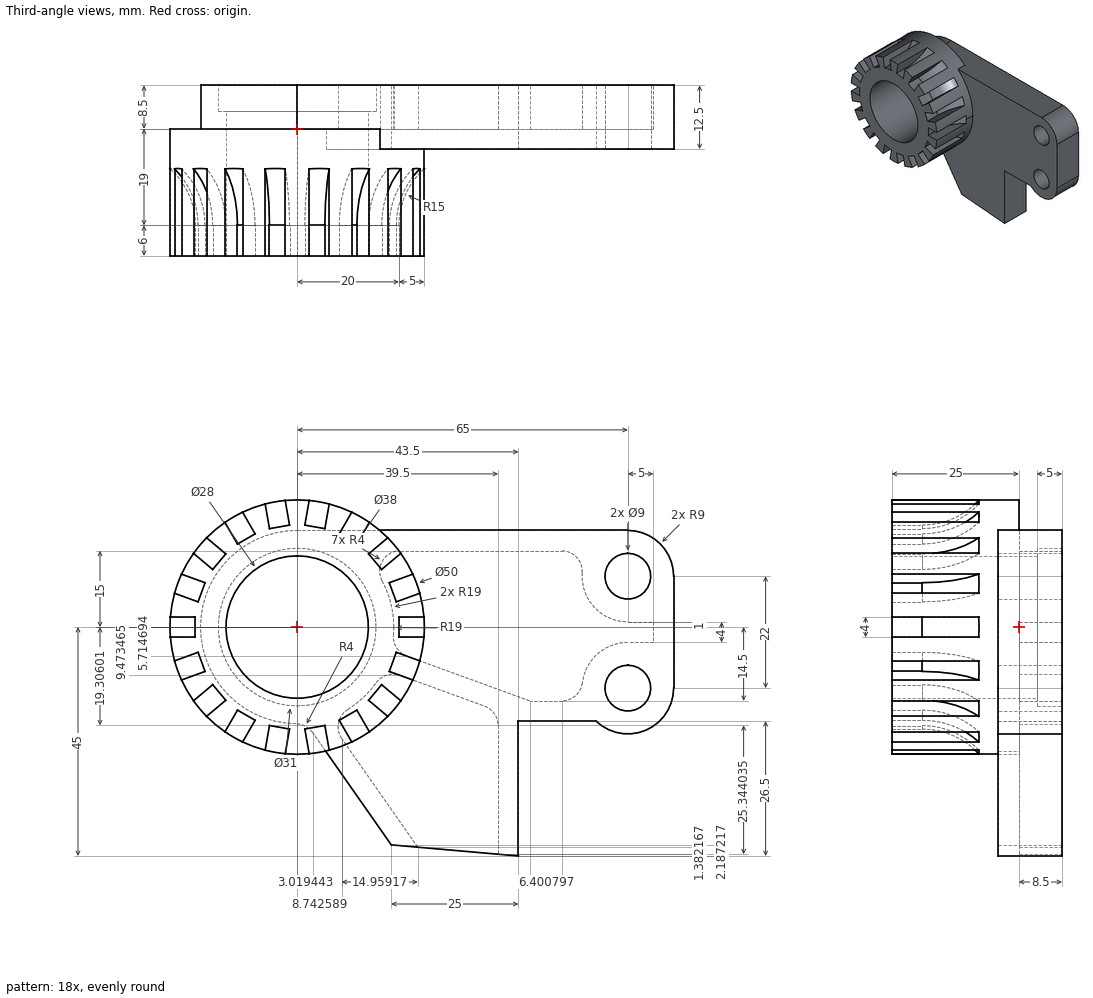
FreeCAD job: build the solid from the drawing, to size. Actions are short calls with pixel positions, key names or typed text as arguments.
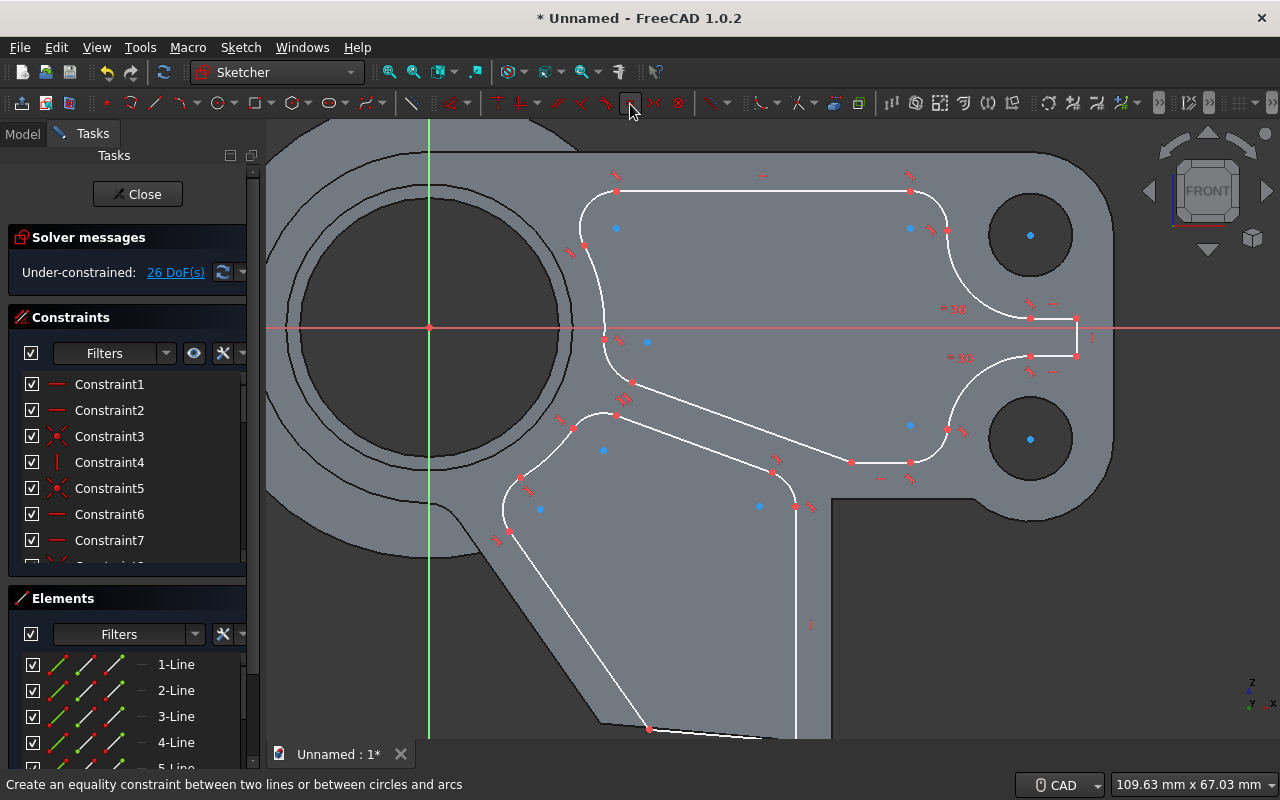
click(944, 213)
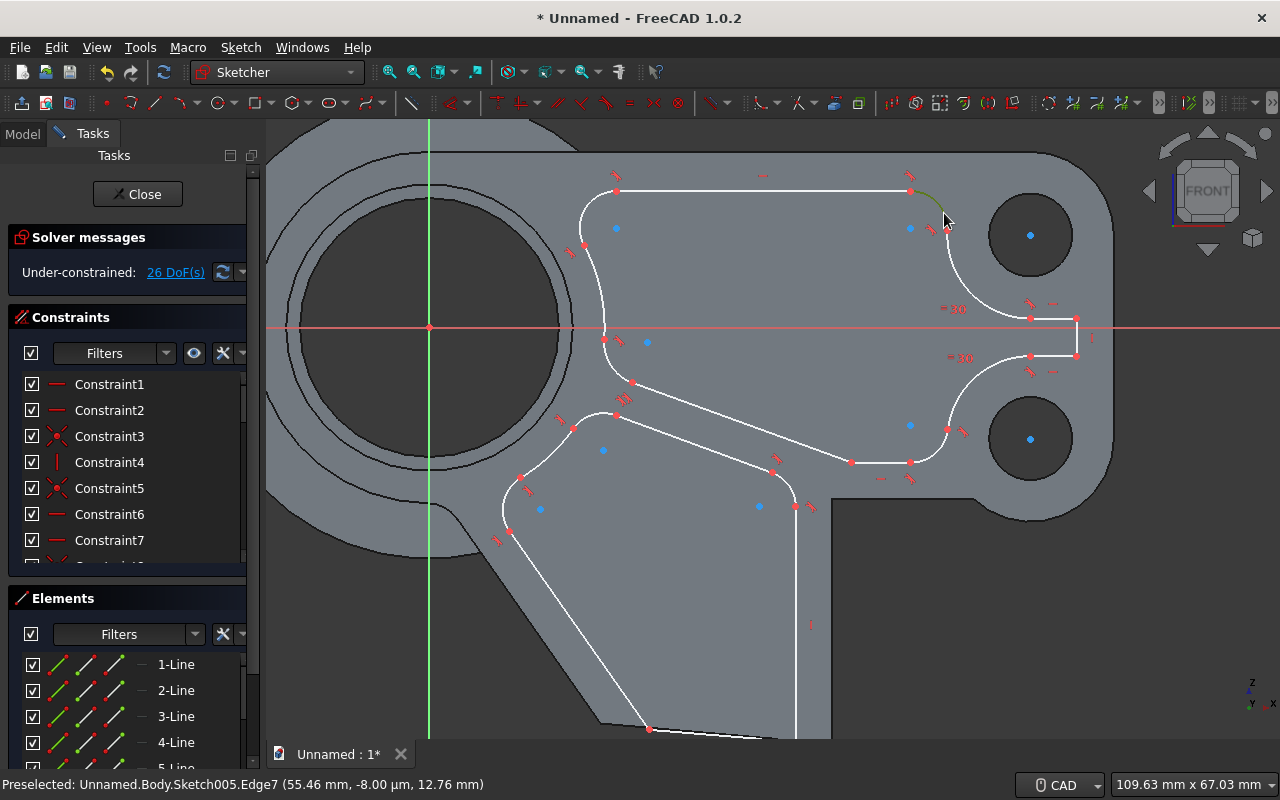
click(927, 459)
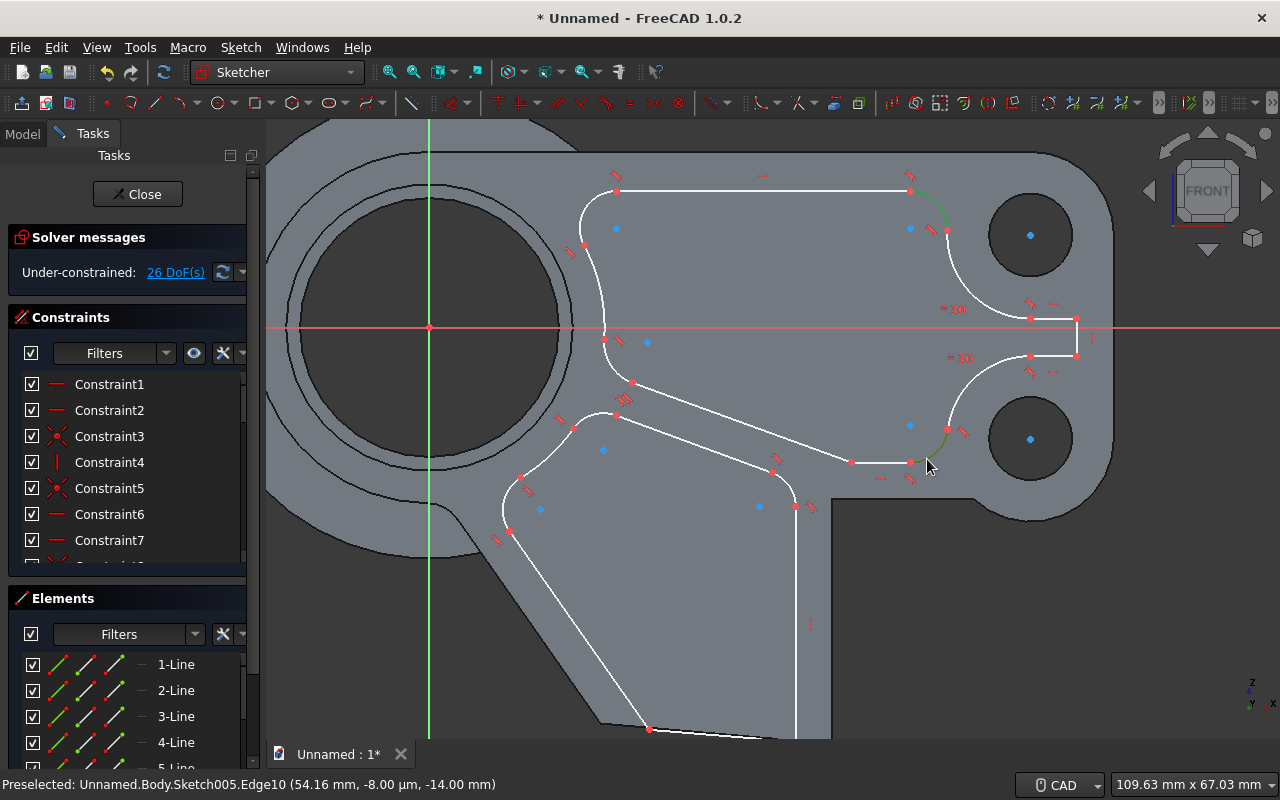
click(606, 356)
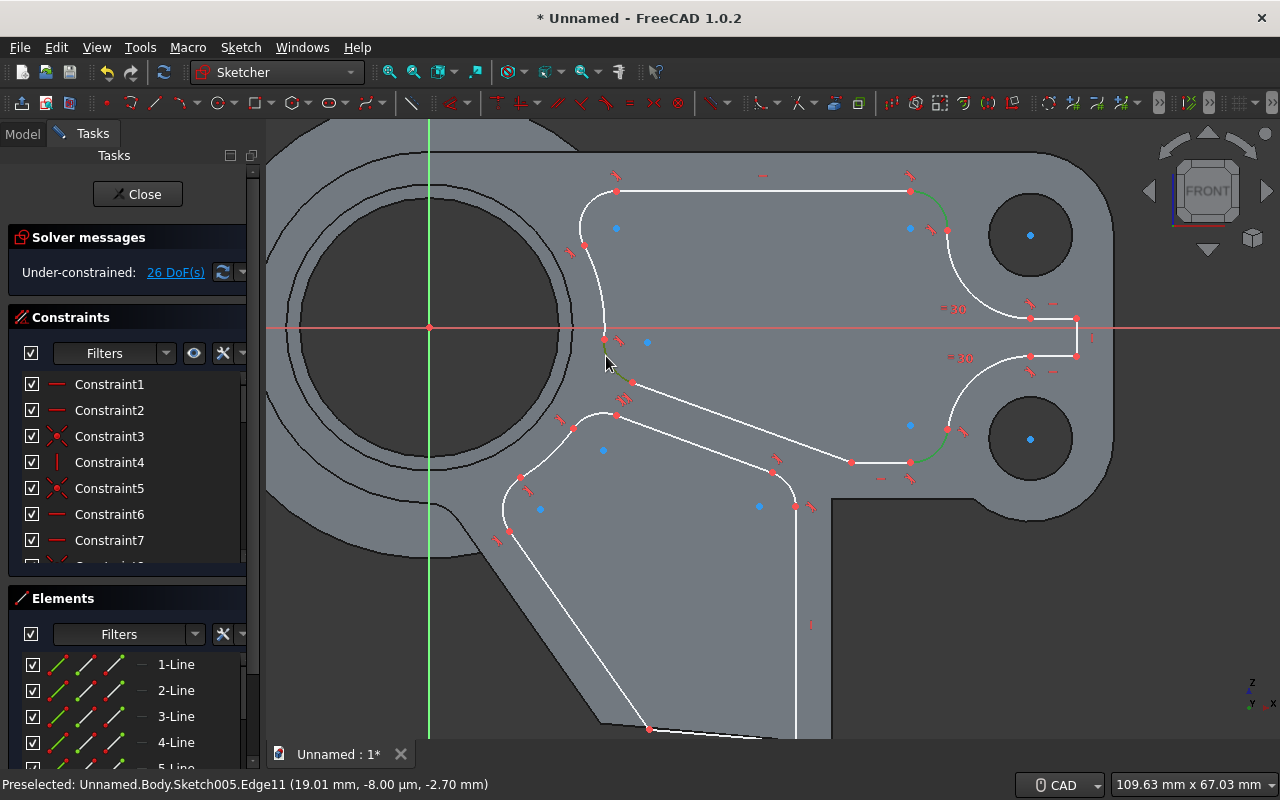
click(595, 198)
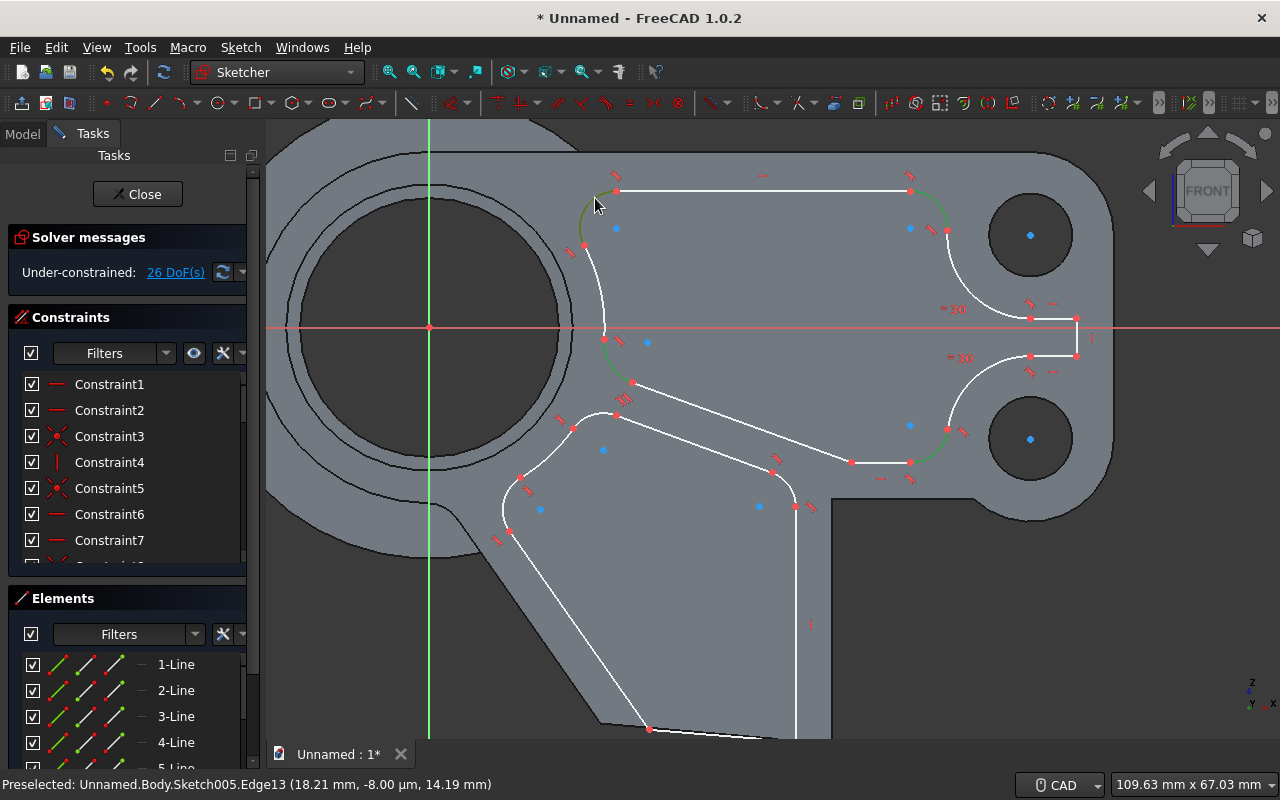
click(793, 494)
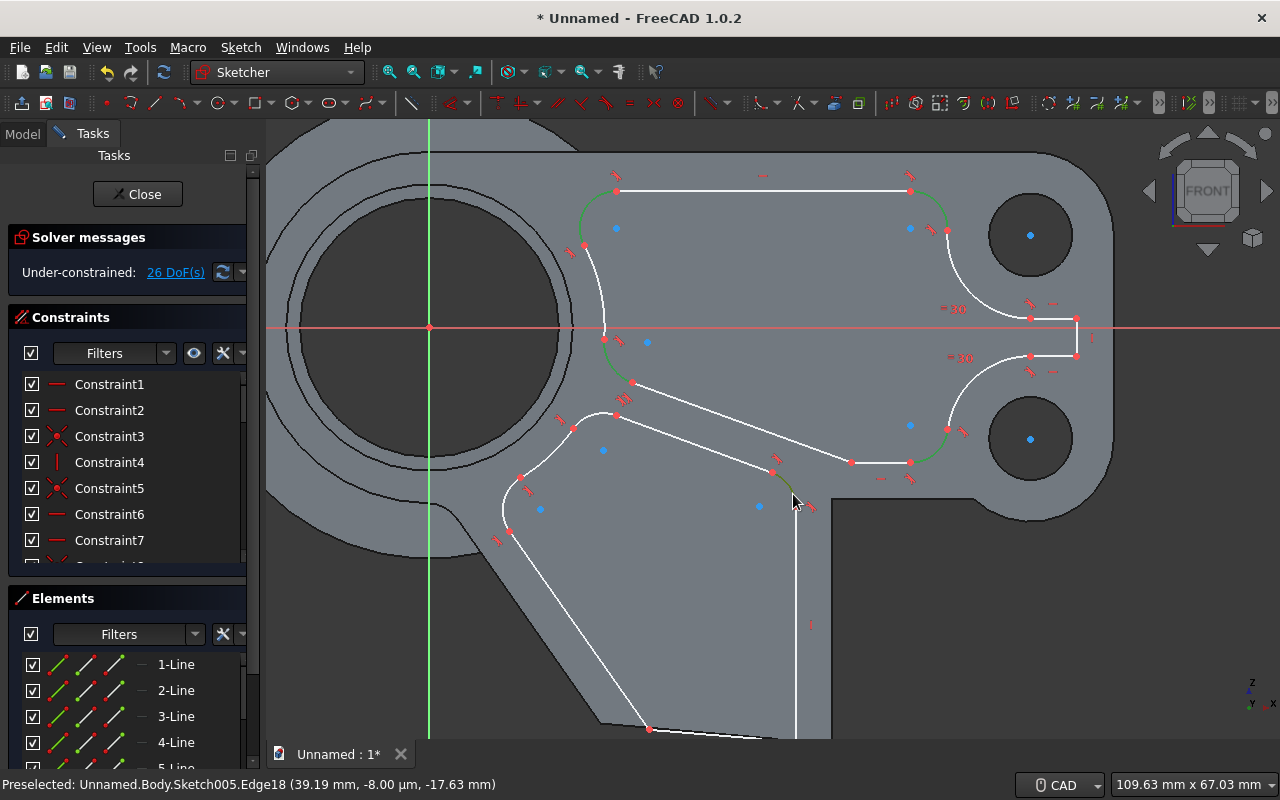
click(508, 491)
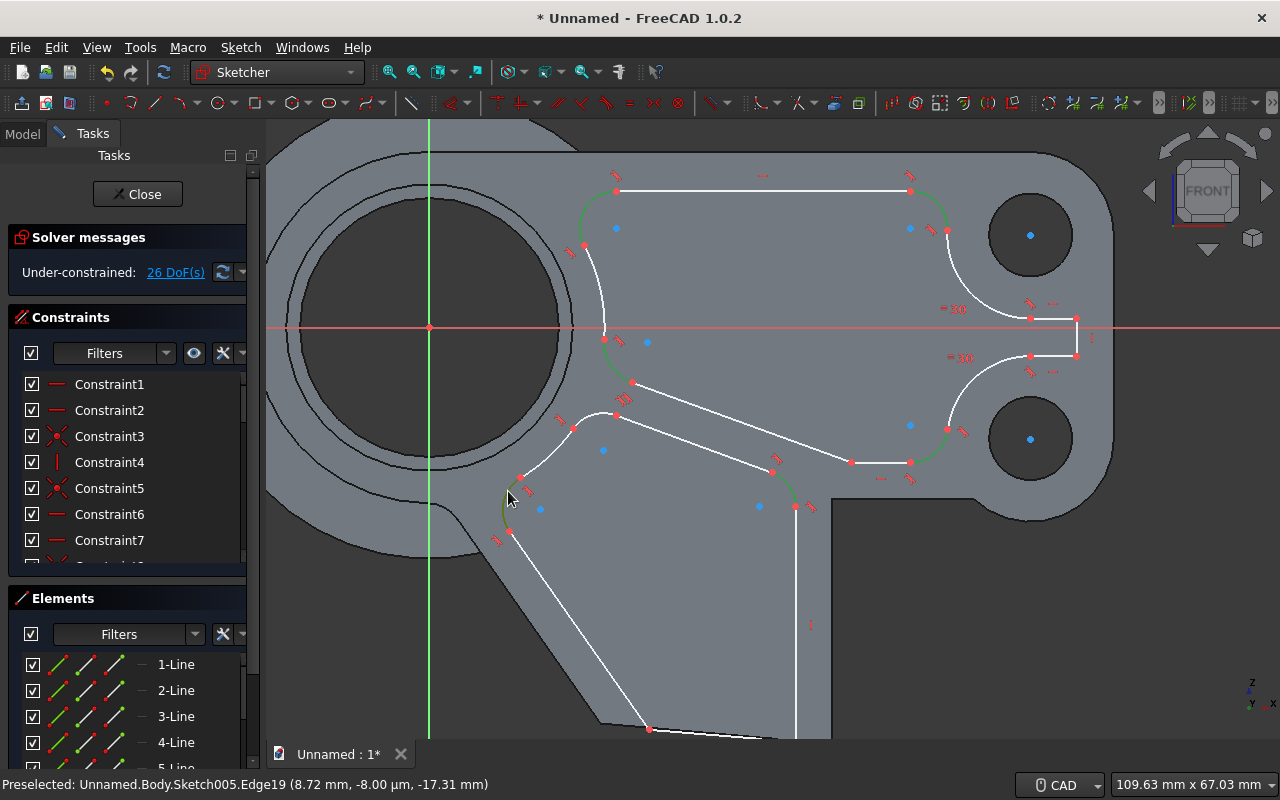
click(602, 413)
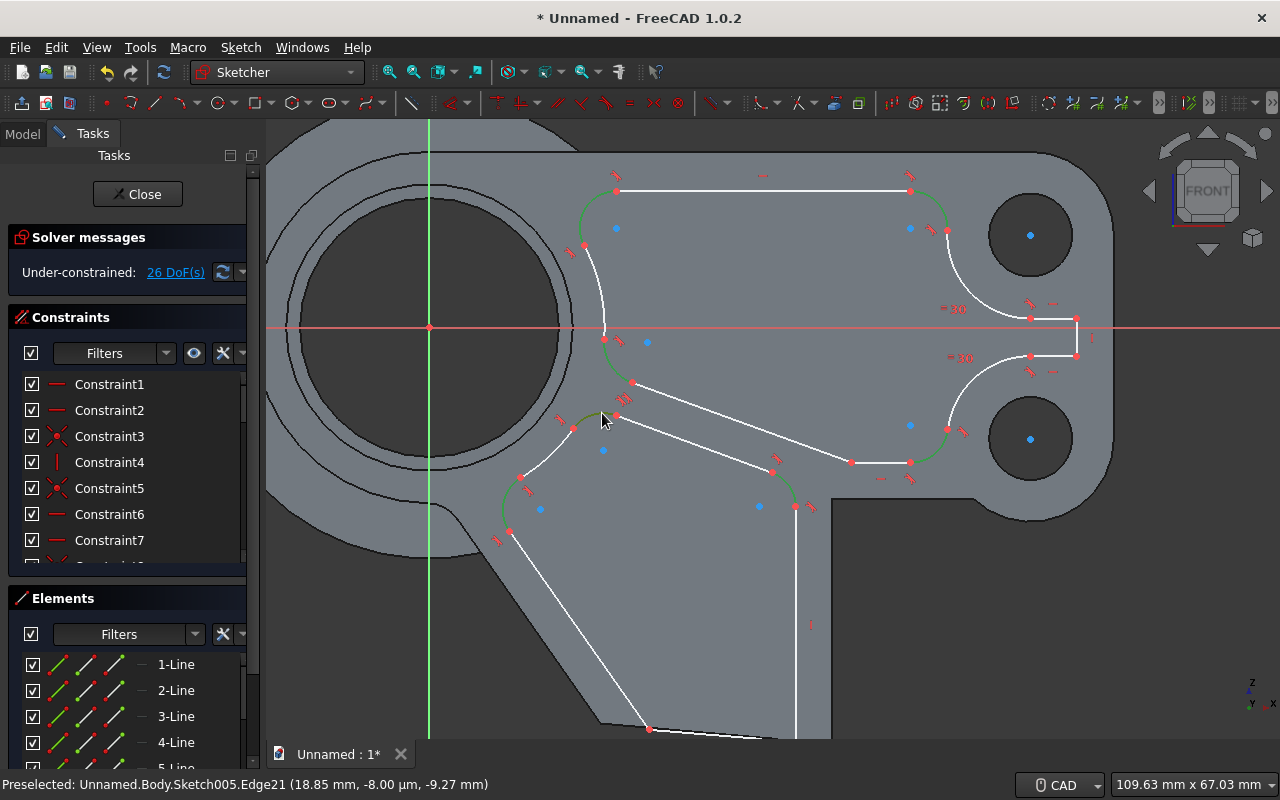
click(630, 104)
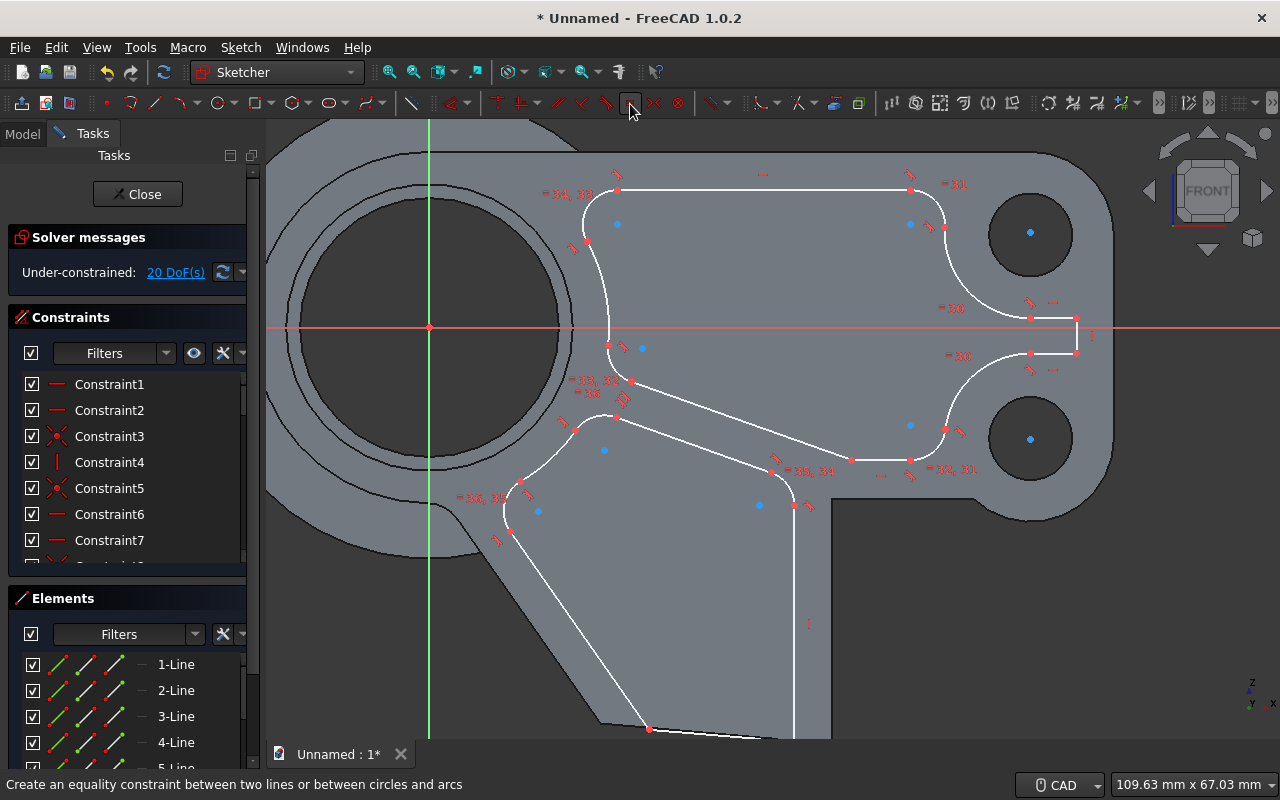
click(450, 104)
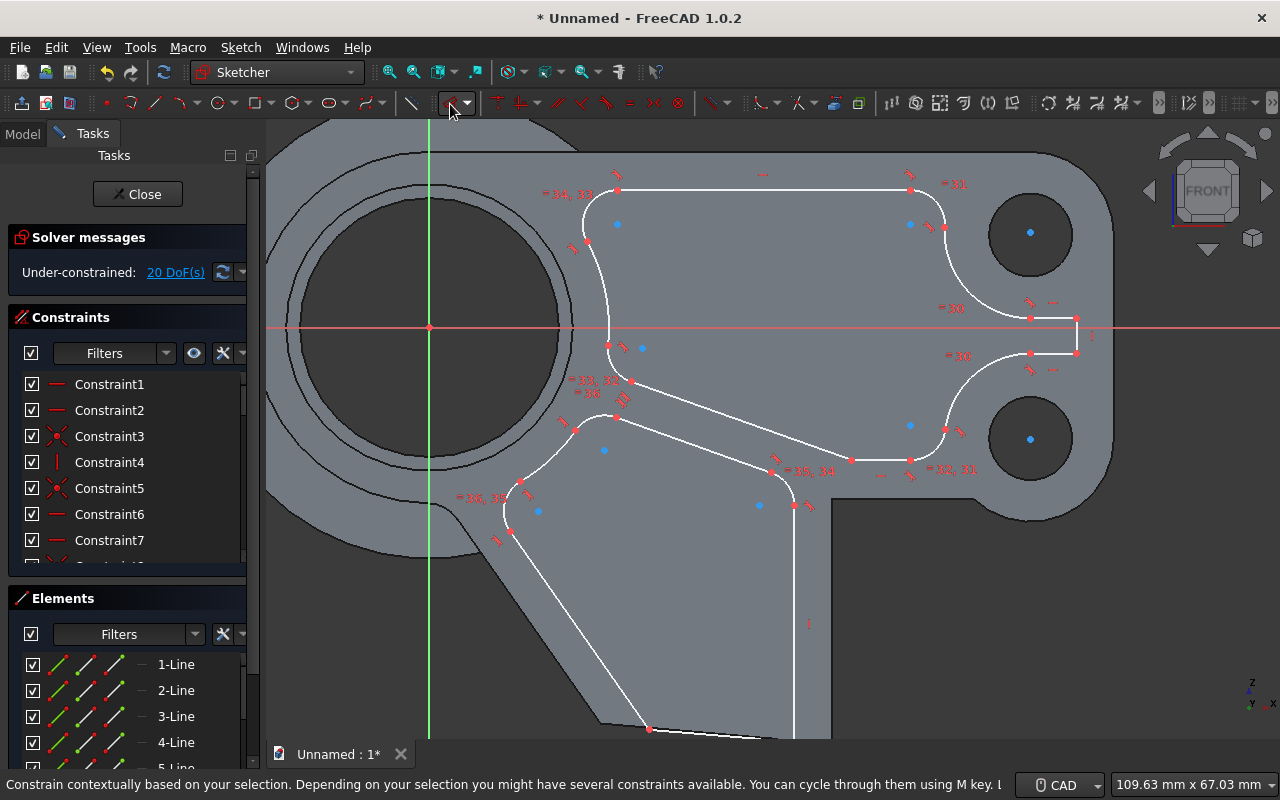
click(942, 210)
click(971, 196)